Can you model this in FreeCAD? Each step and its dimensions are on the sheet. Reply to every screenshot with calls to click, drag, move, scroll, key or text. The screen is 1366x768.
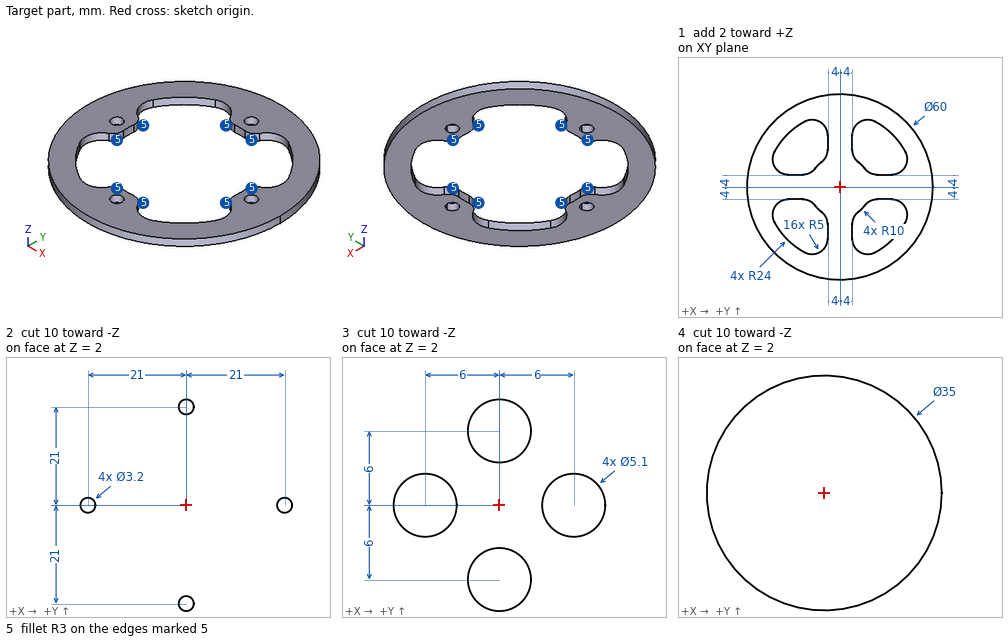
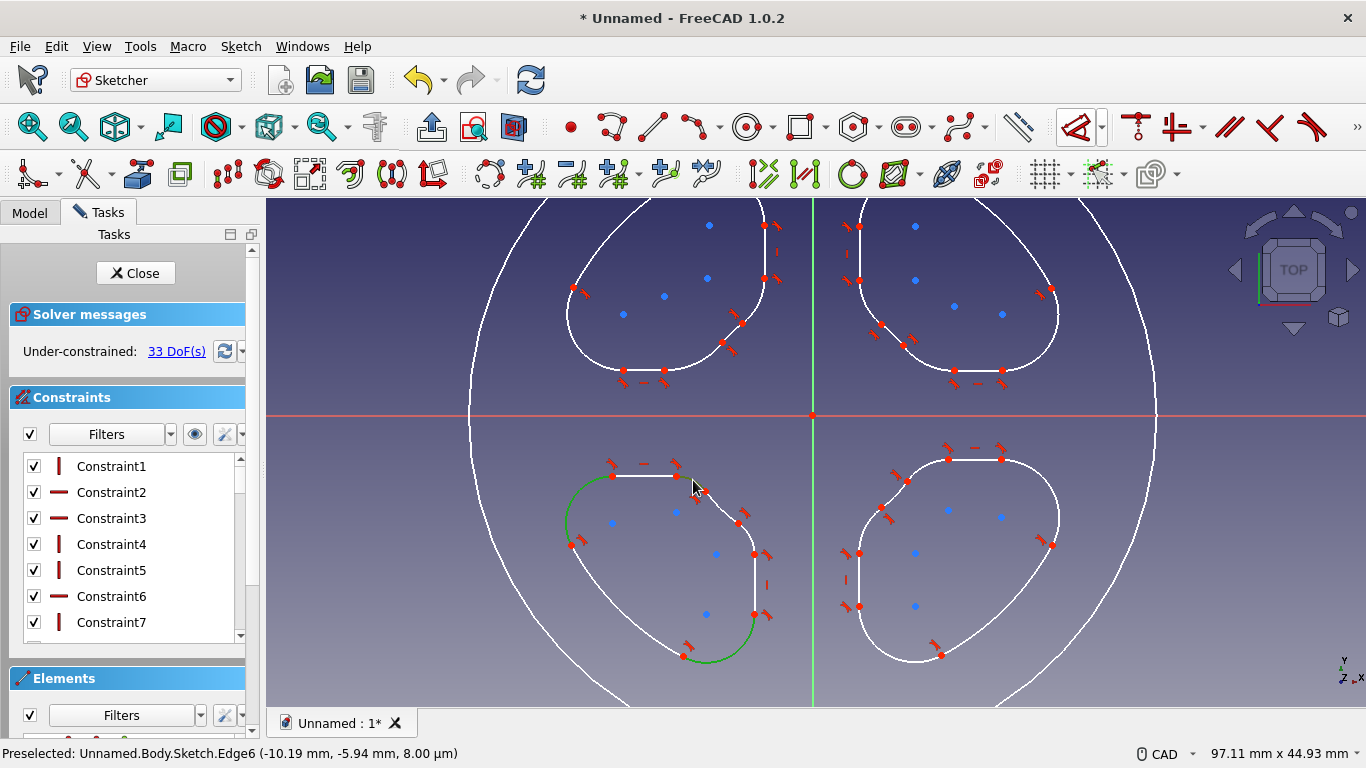
scroll(753, 544, up, 2)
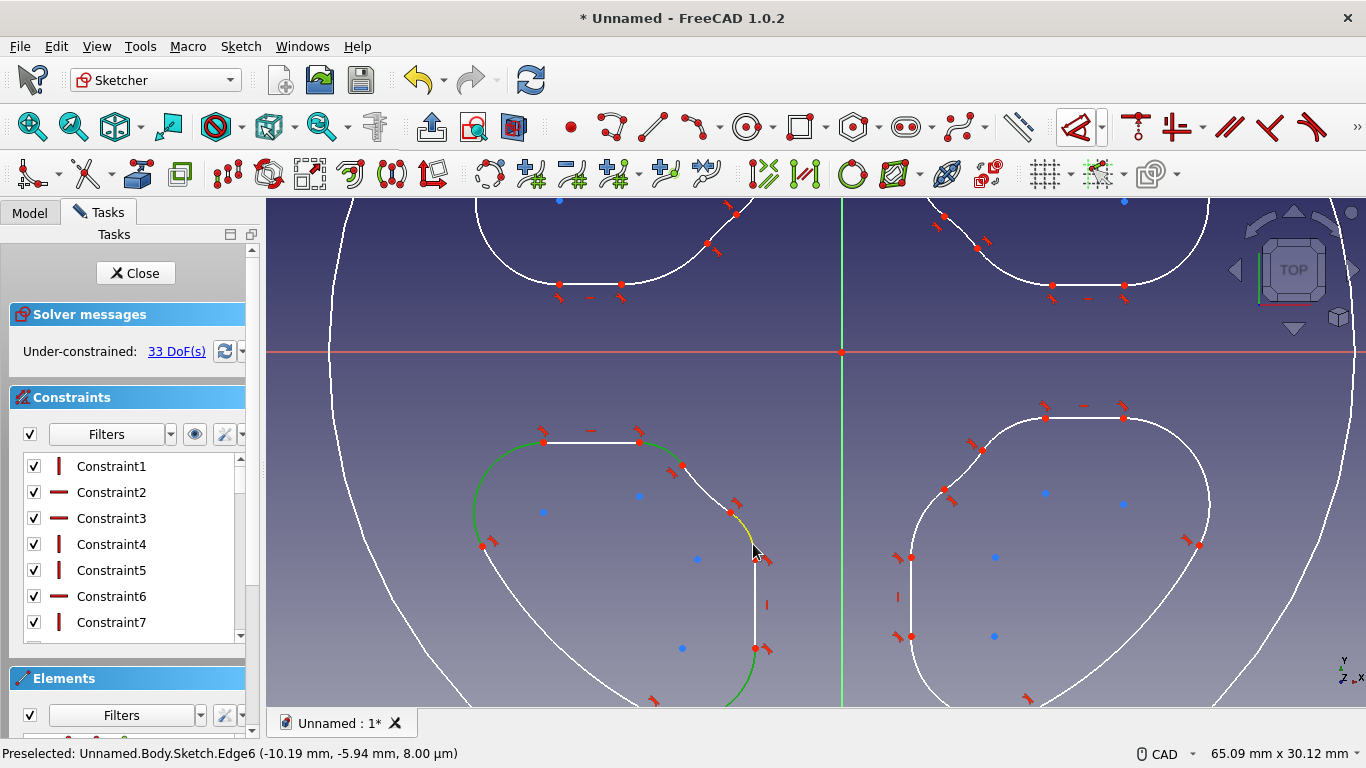
click(753, 543)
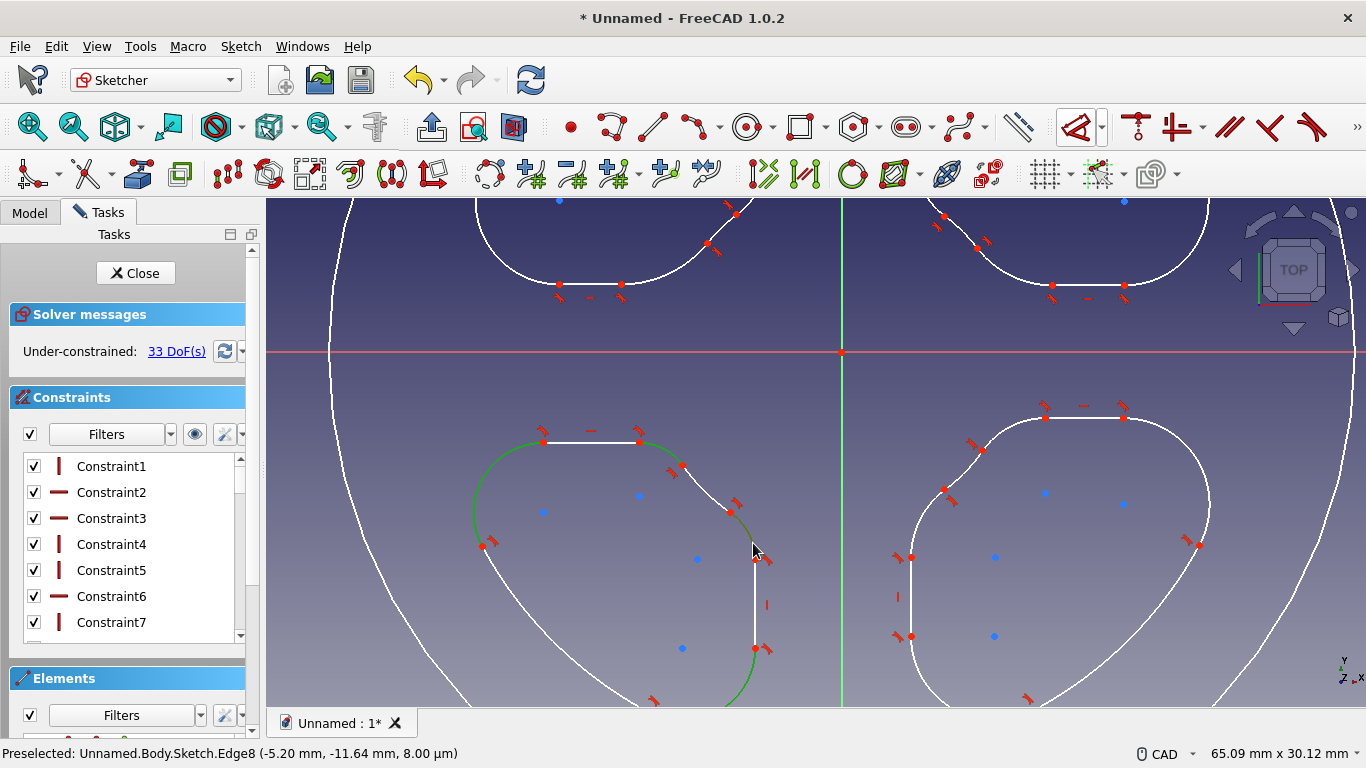
click(1173, 434)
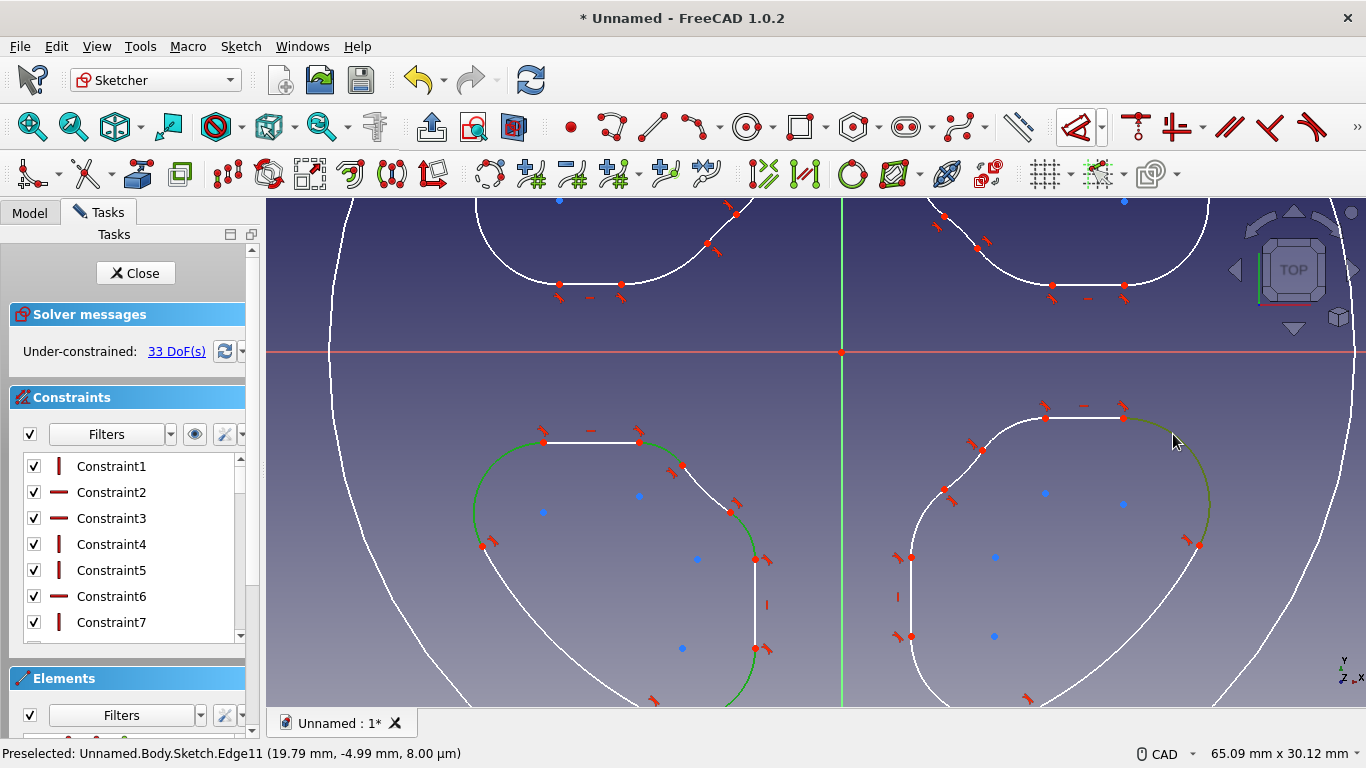
click(918, 670)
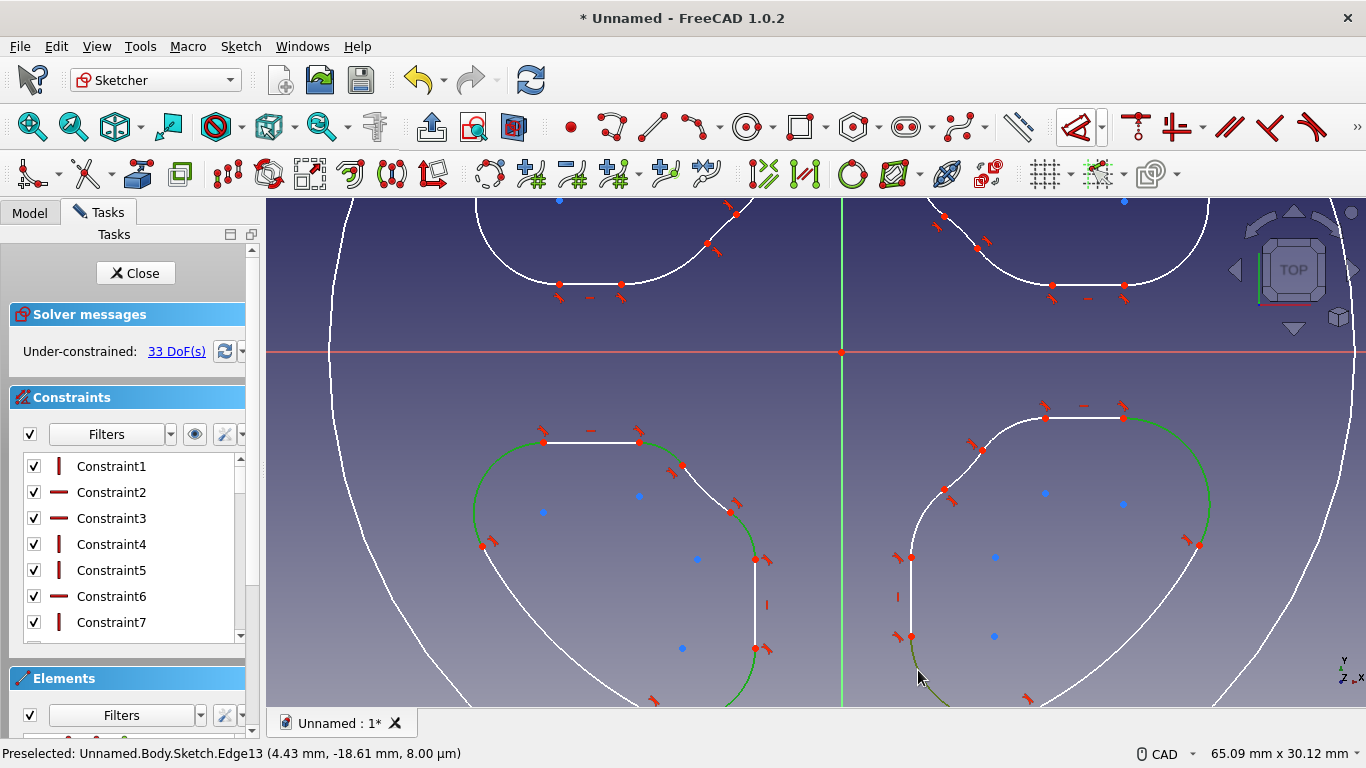
click(928, 506)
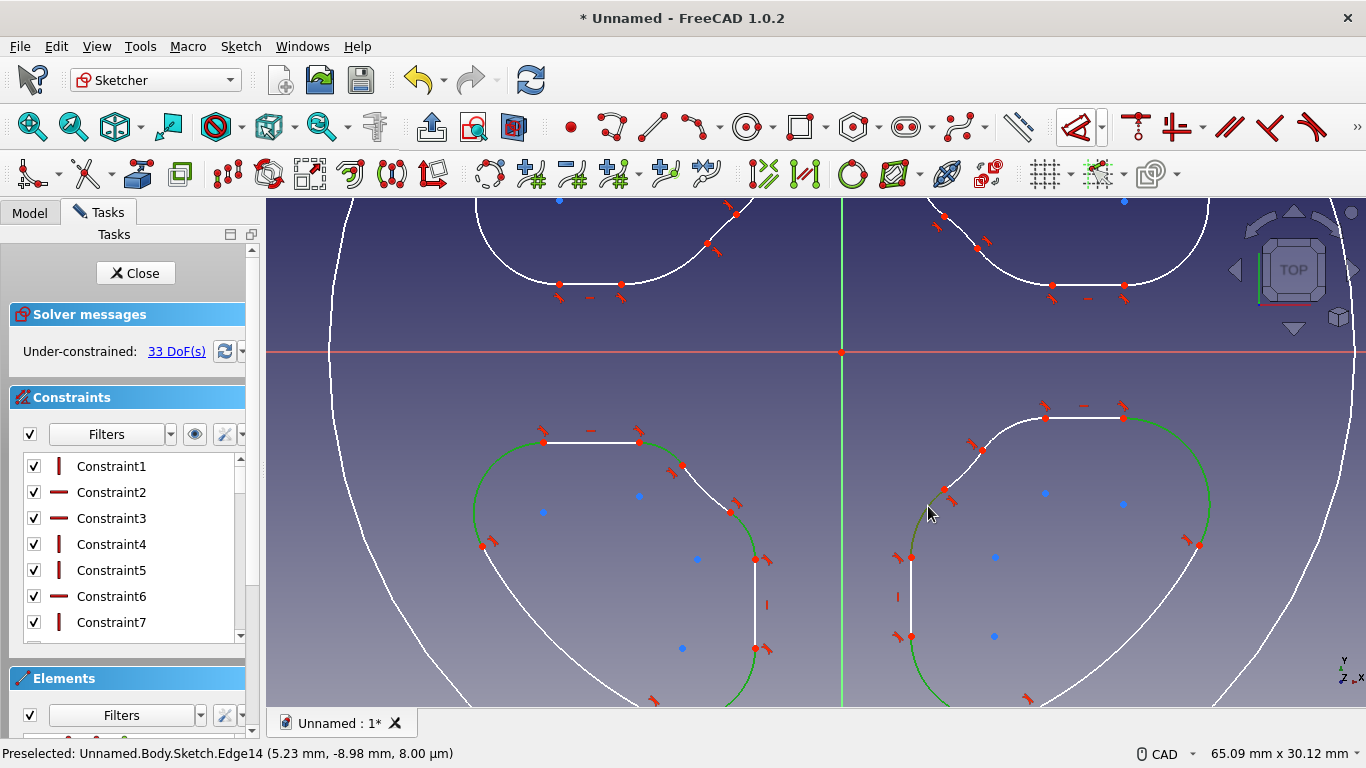
click(1024, 421)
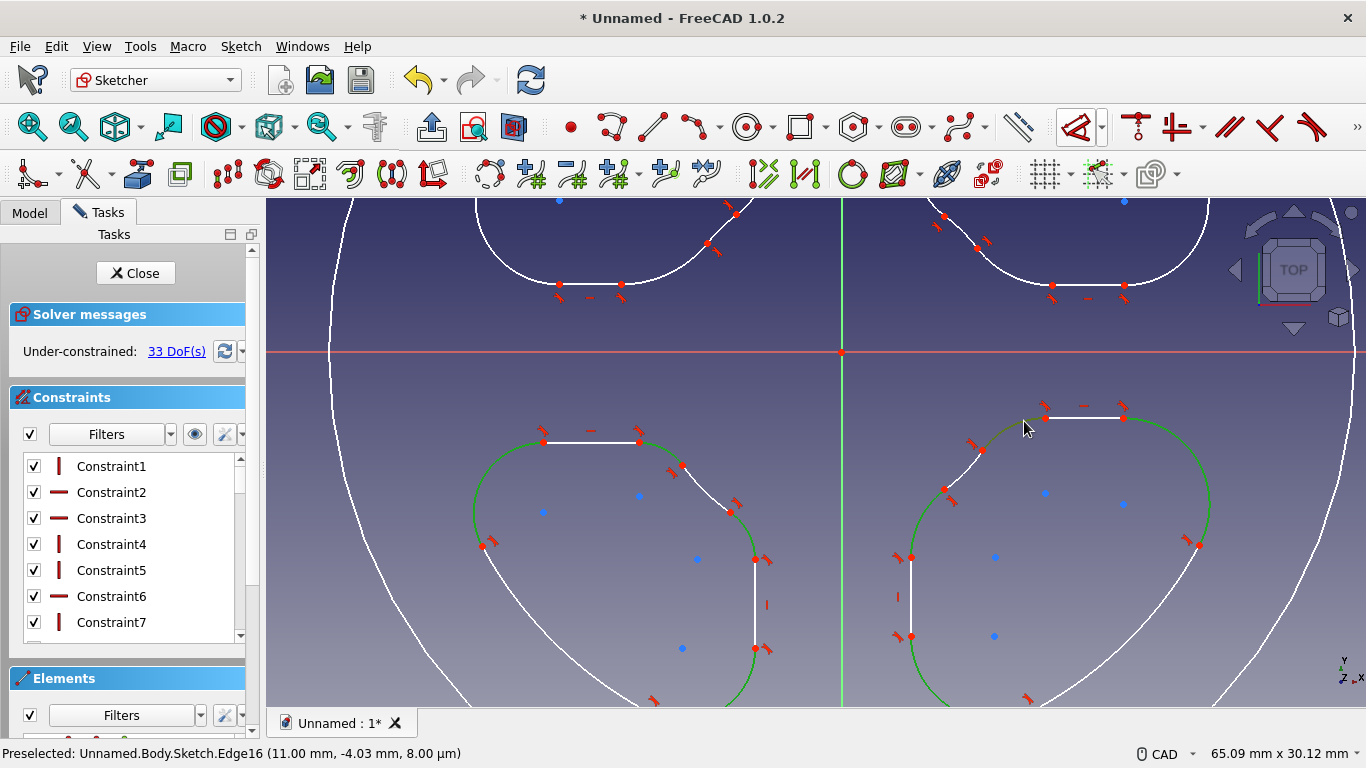
scroll(707, 496, down, 6)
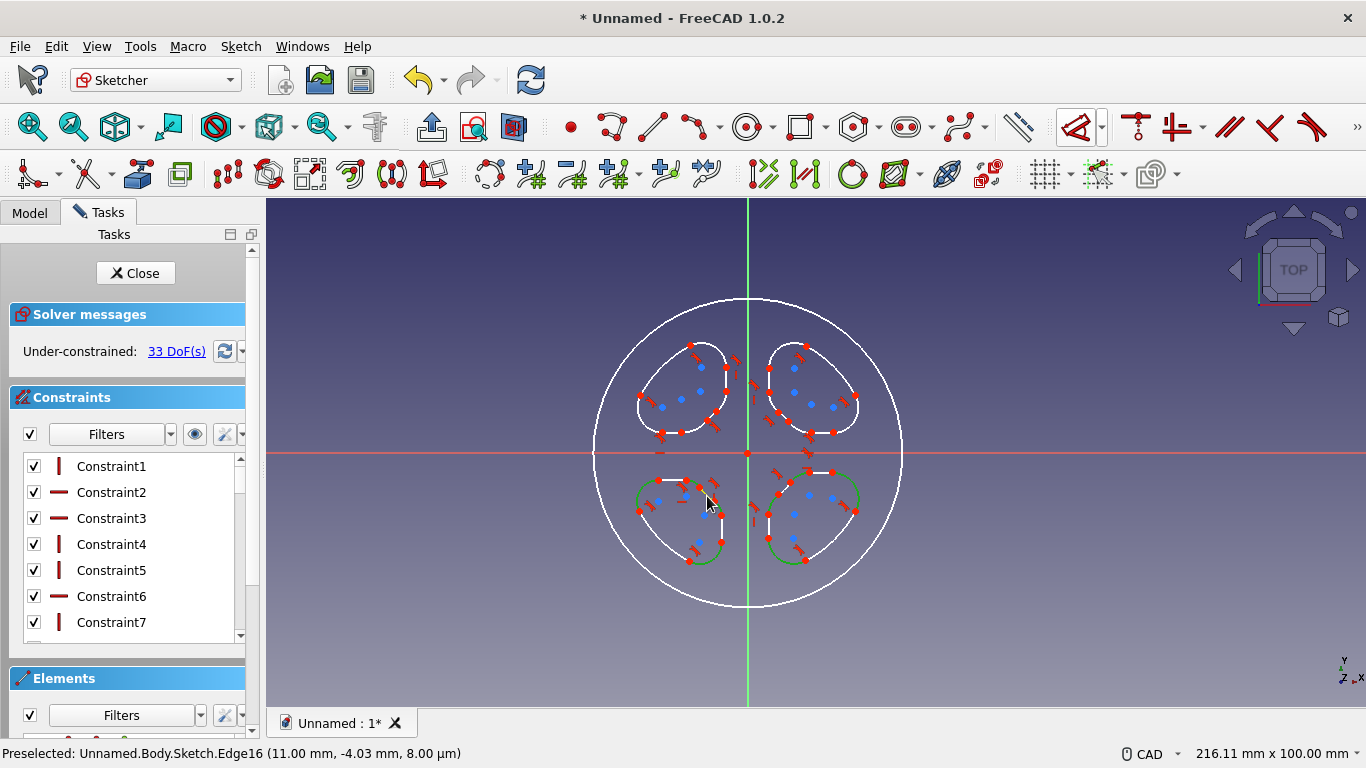
scroll(721, 407, up, 4)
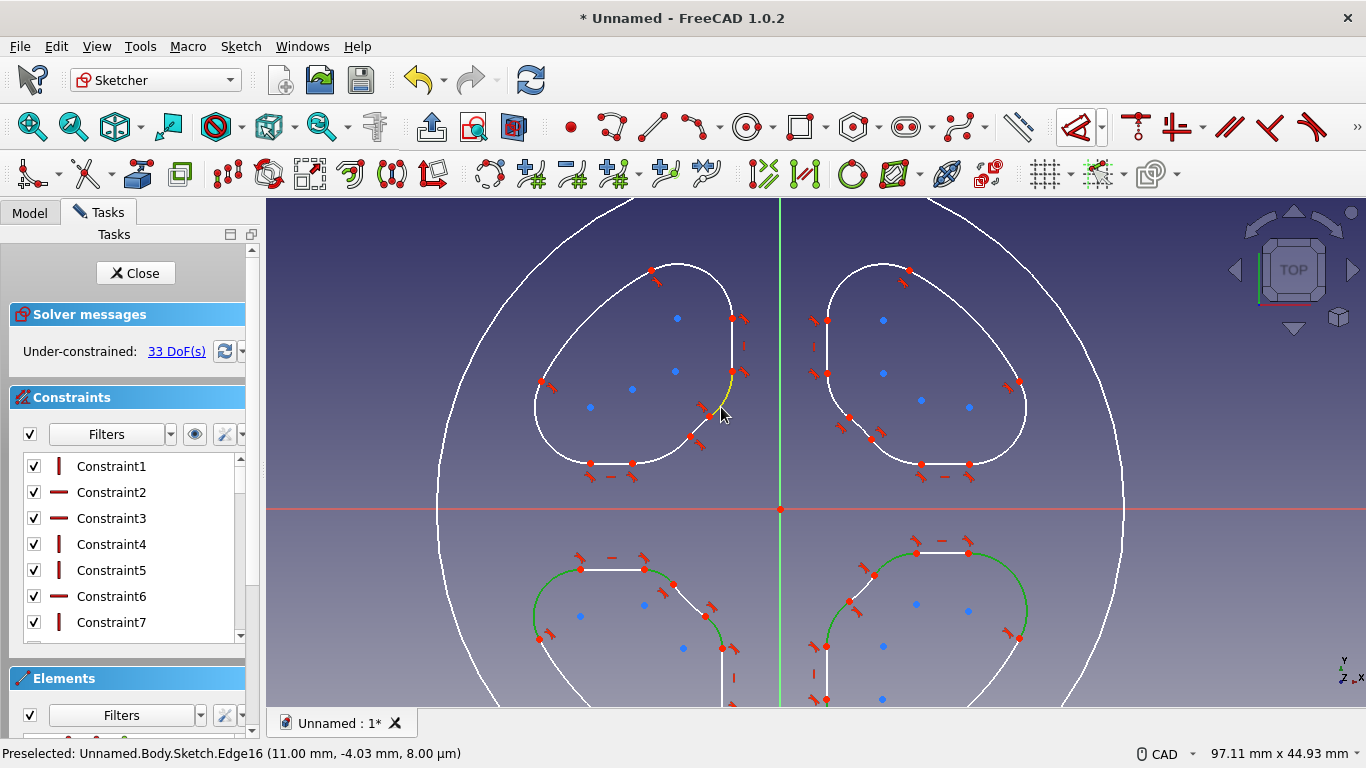
click(721, 406)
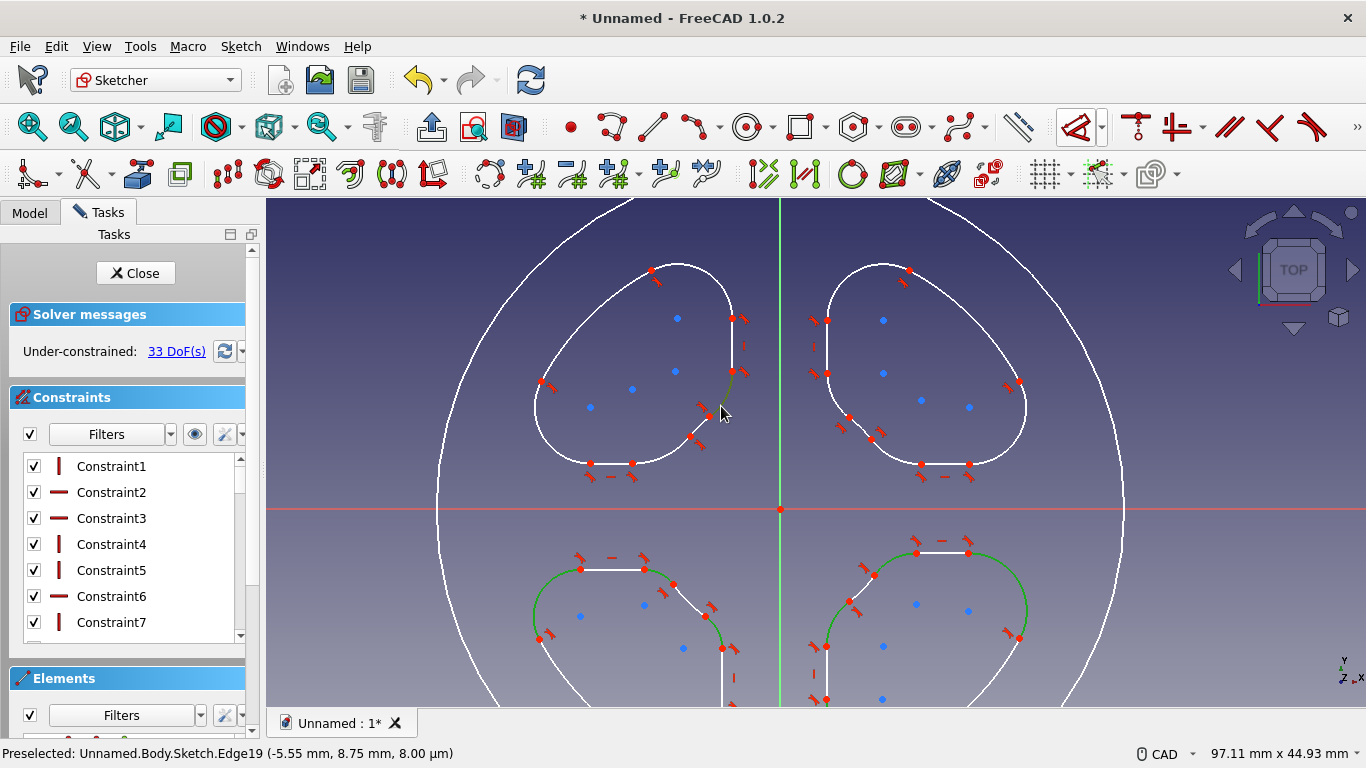
click(652, 461)